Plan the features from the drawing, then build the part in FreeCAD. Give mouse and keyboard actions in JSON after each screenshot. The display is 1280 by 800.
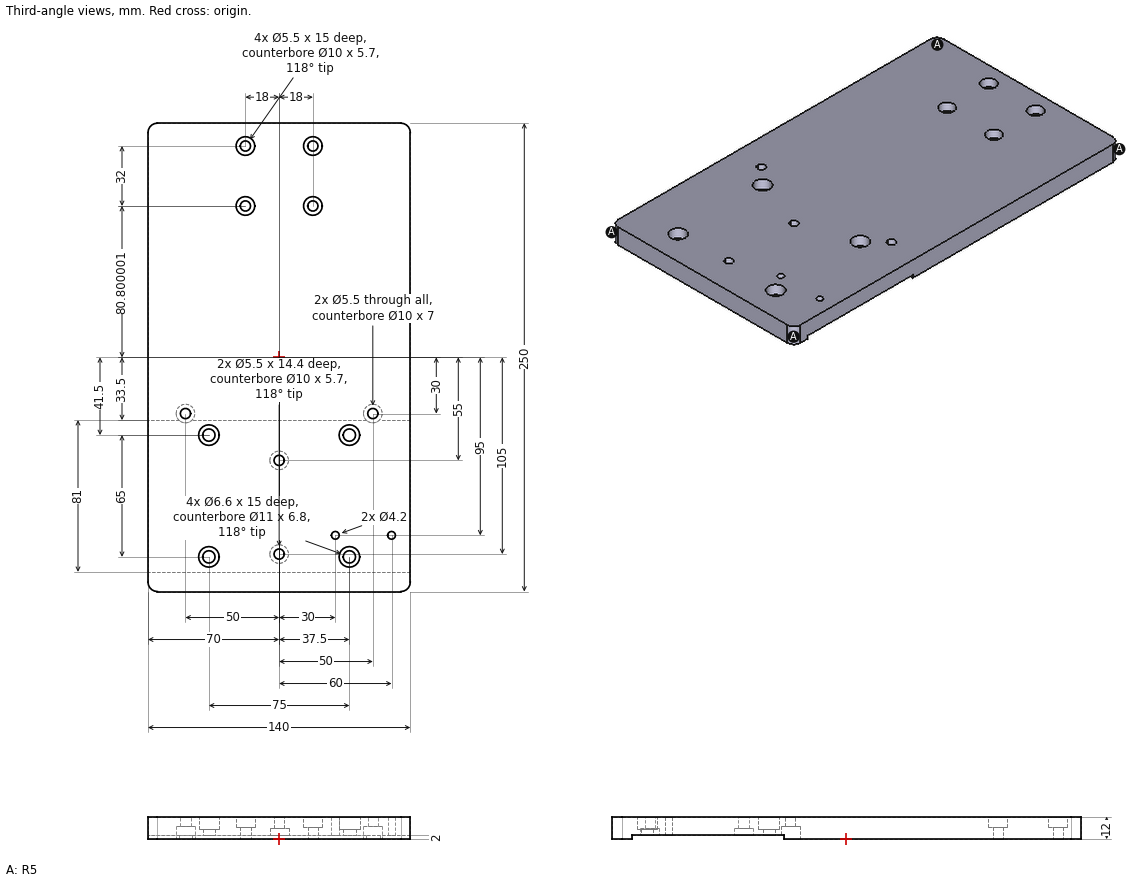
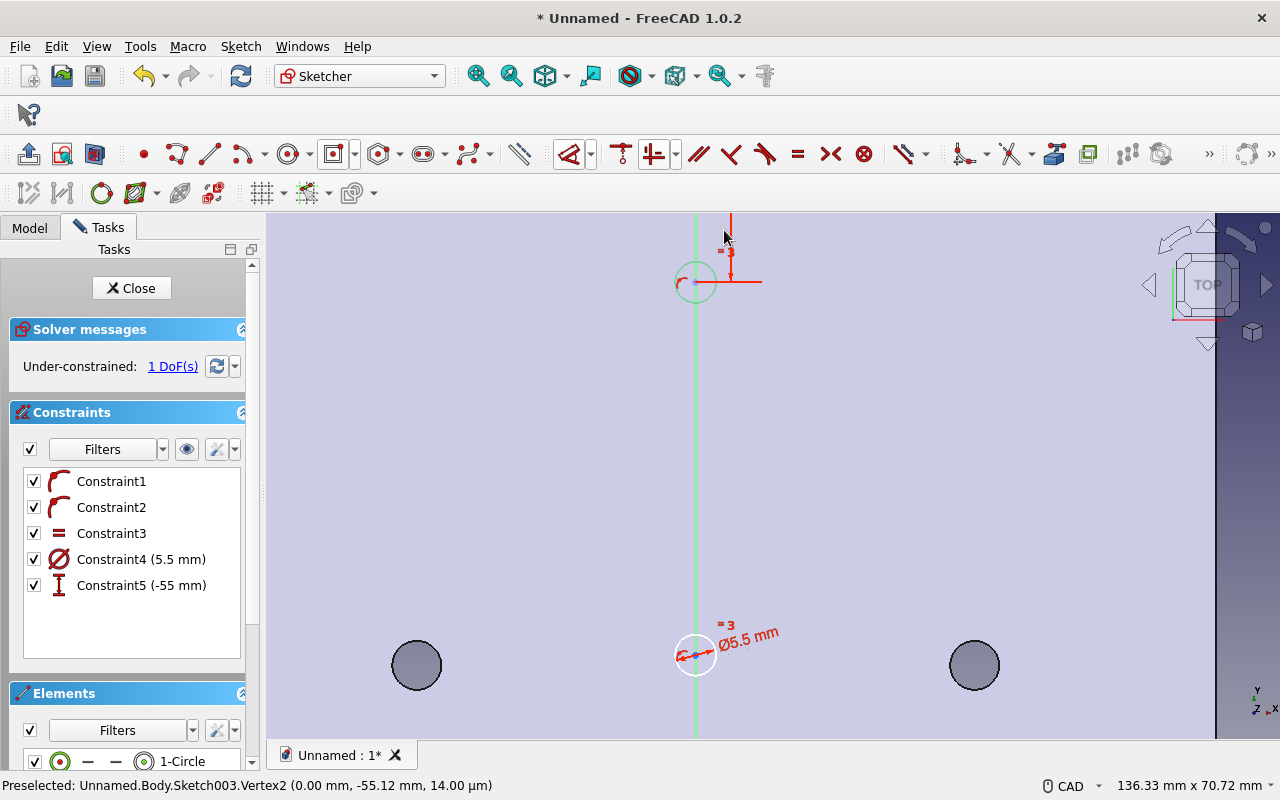
{"action": "left_click", "coordinate": [696, 655]}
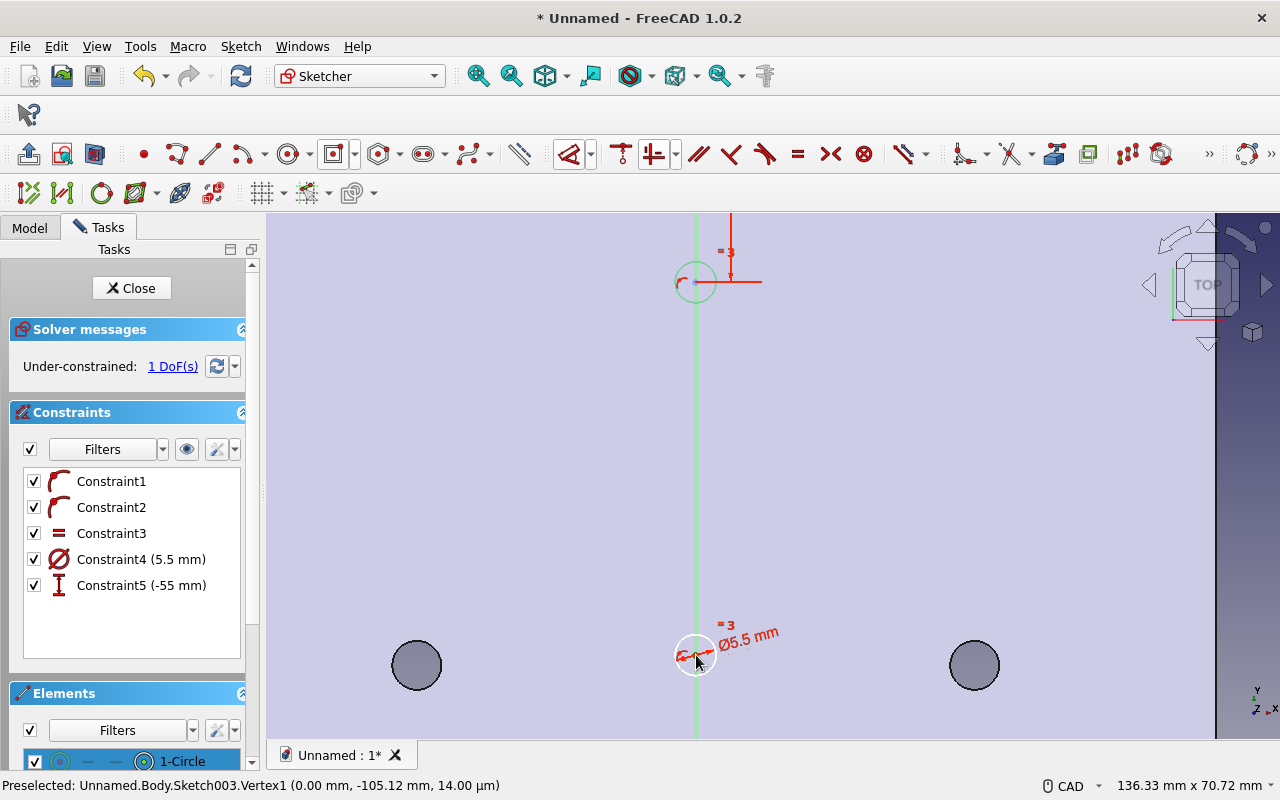
{"action": "key", "text": "i"}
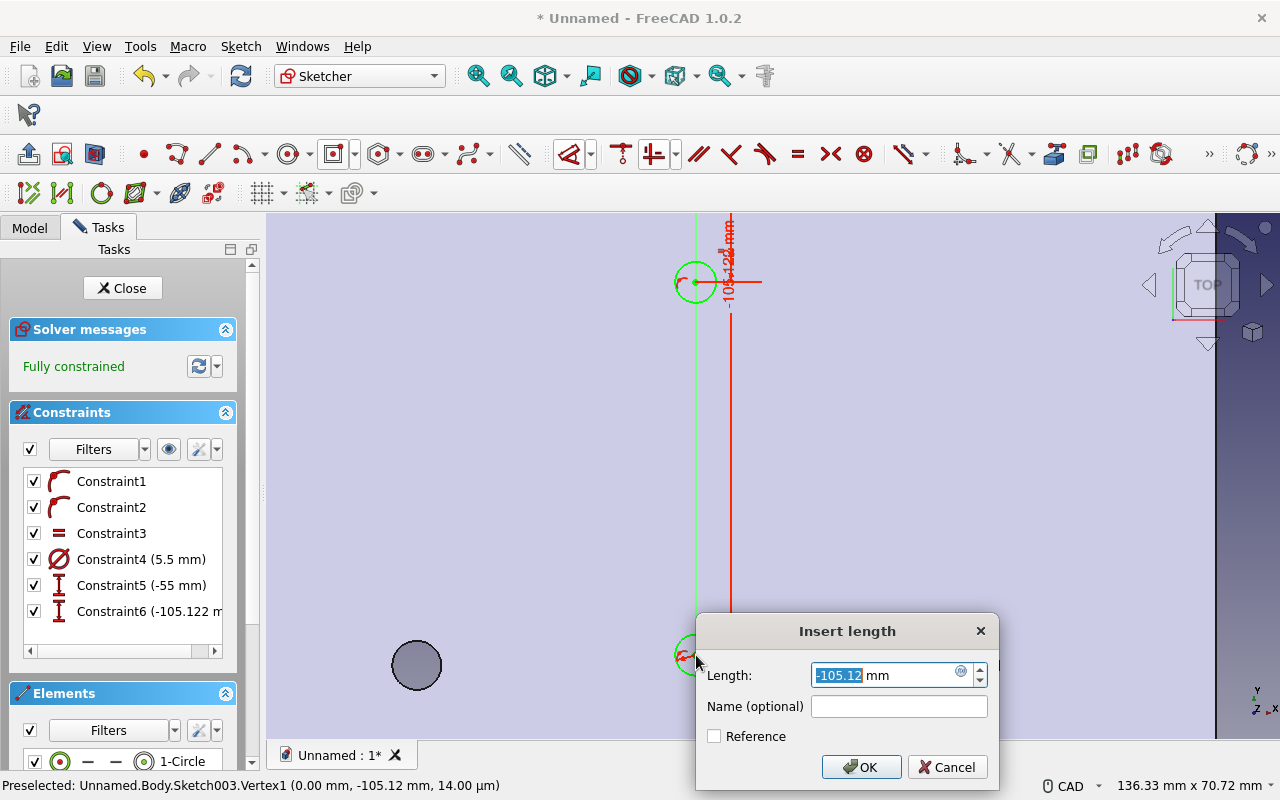
{"action": "type", "text": "-105"}
{"action": "key", "text": "Return"}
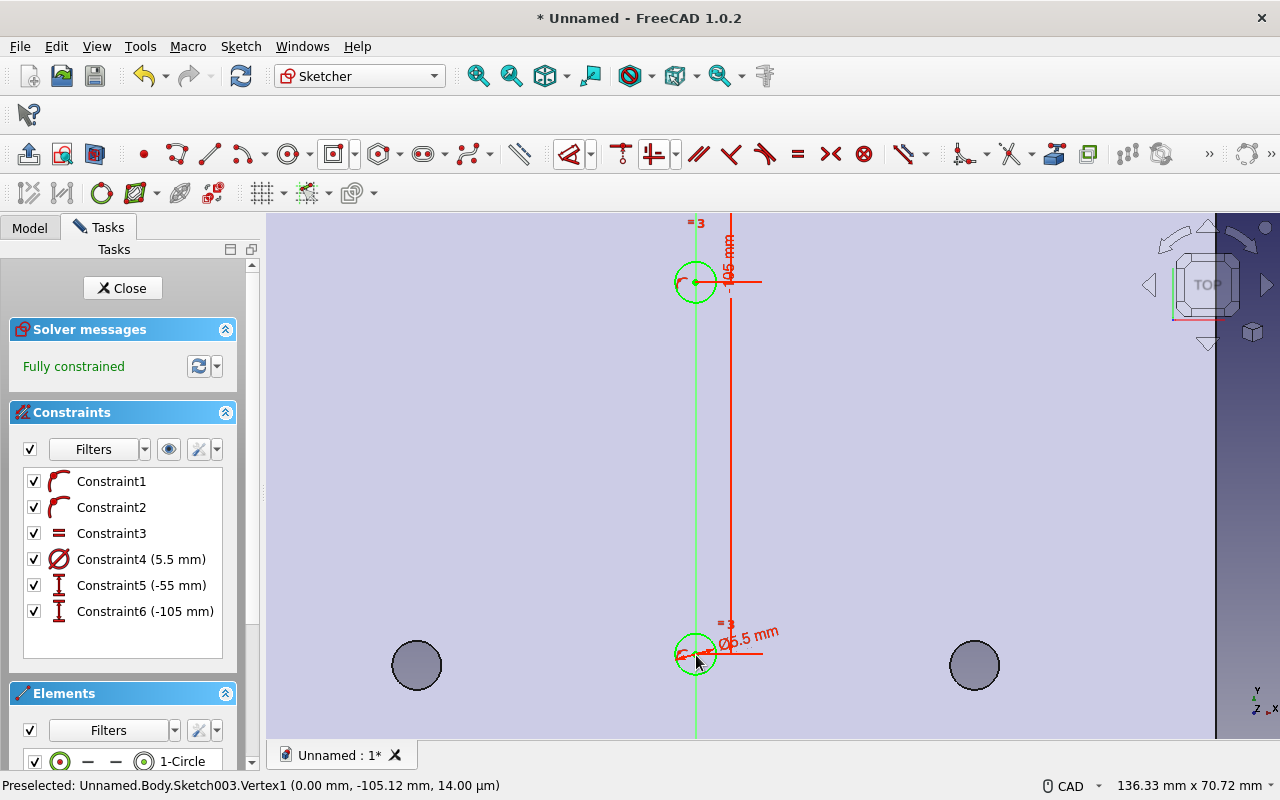
{"action": "left_click", "coordinate": [123, 288]}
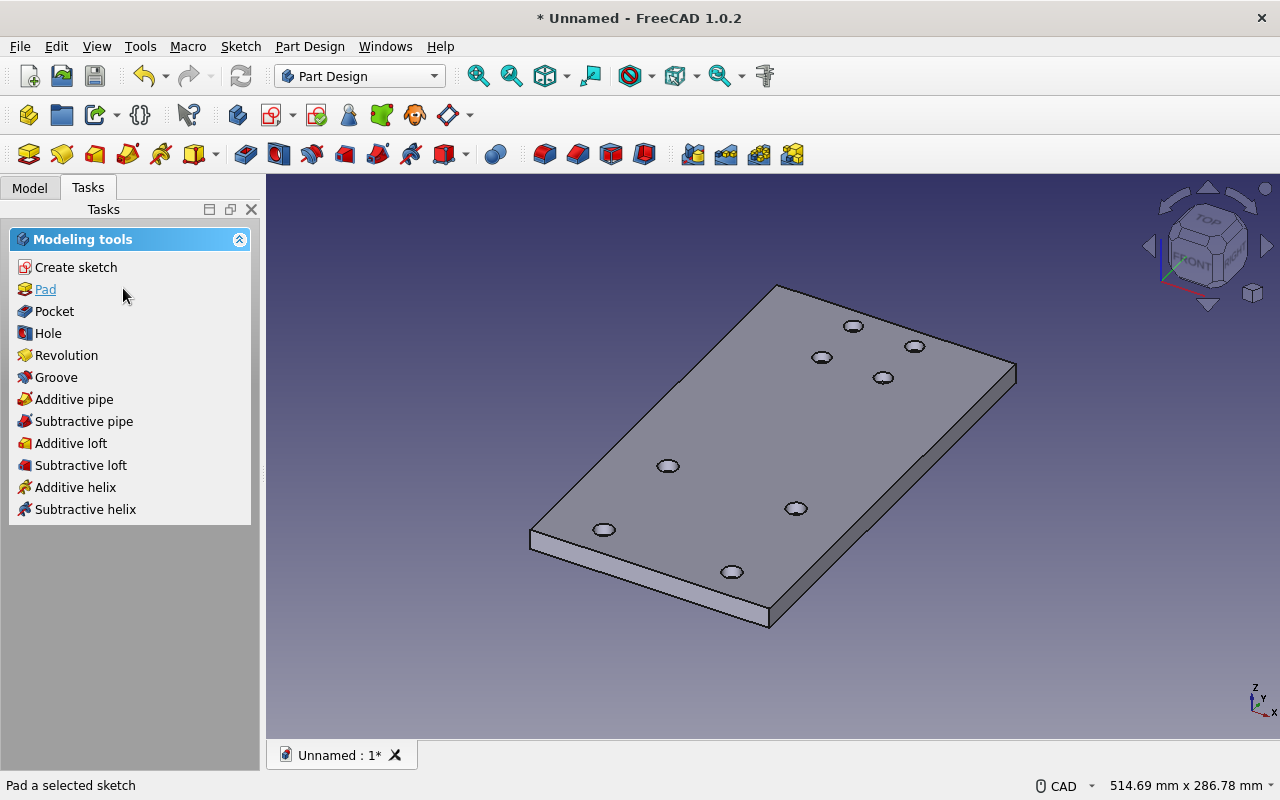
{"action": "left_click", "coordinate": [279, 154]}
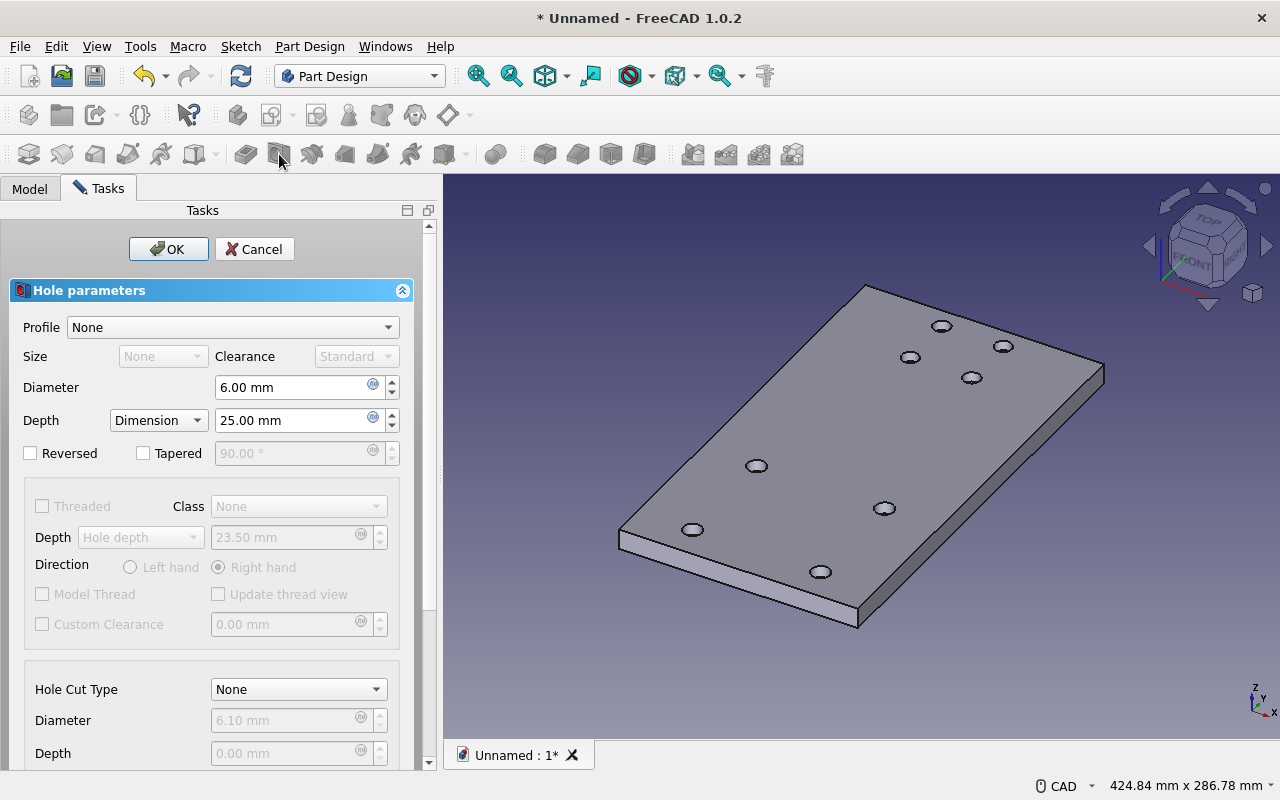
{"action": "triple_click", "coordinate": [300, 388]}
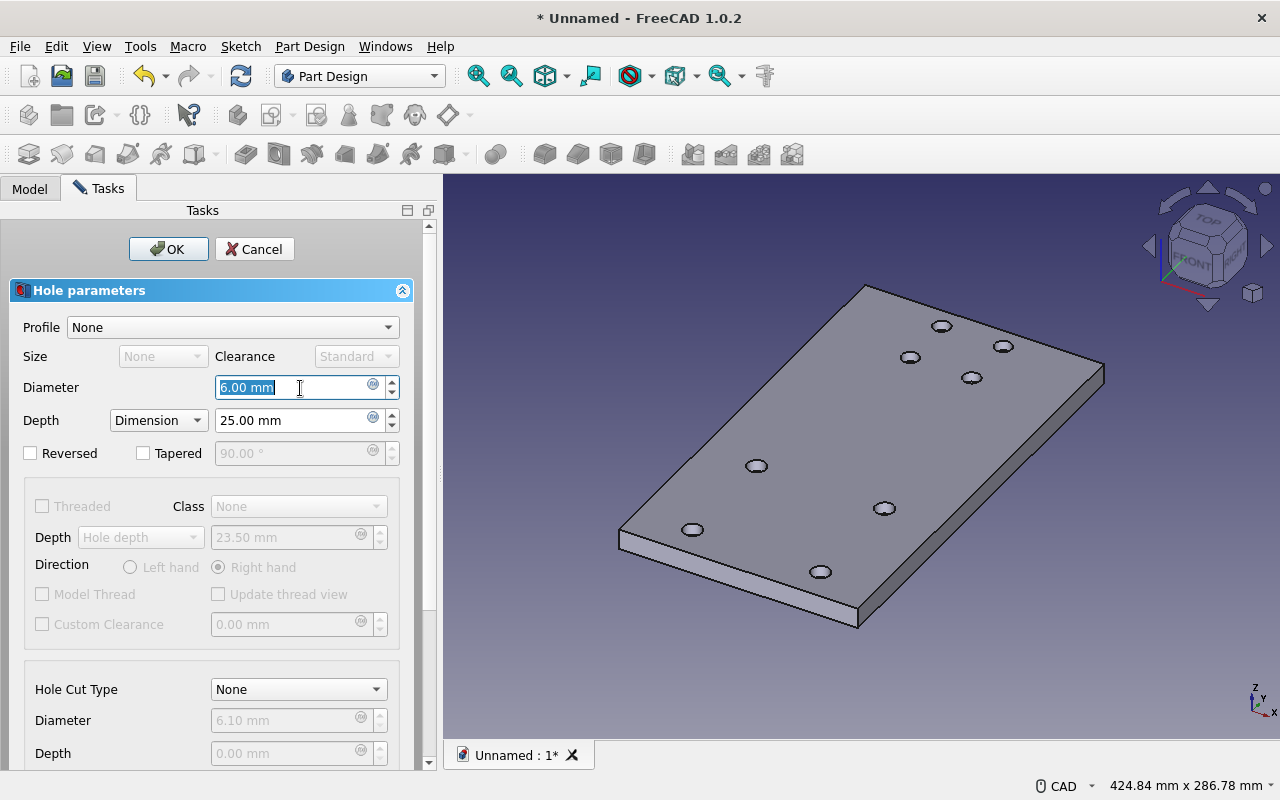
{"action": "type", "text": "5.5"}
{"action": "key", "text": "Tab"}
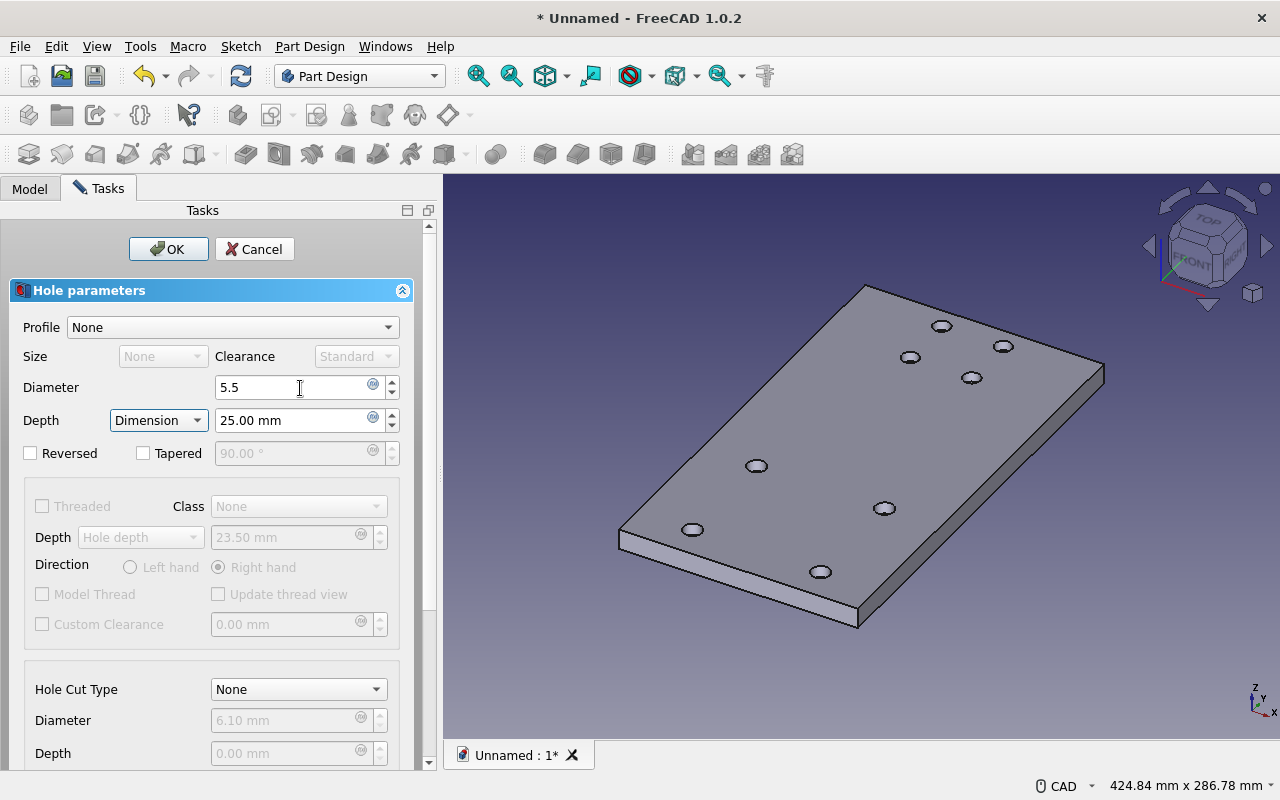
{"action": "triple_click", "coordinate": [300, 420]}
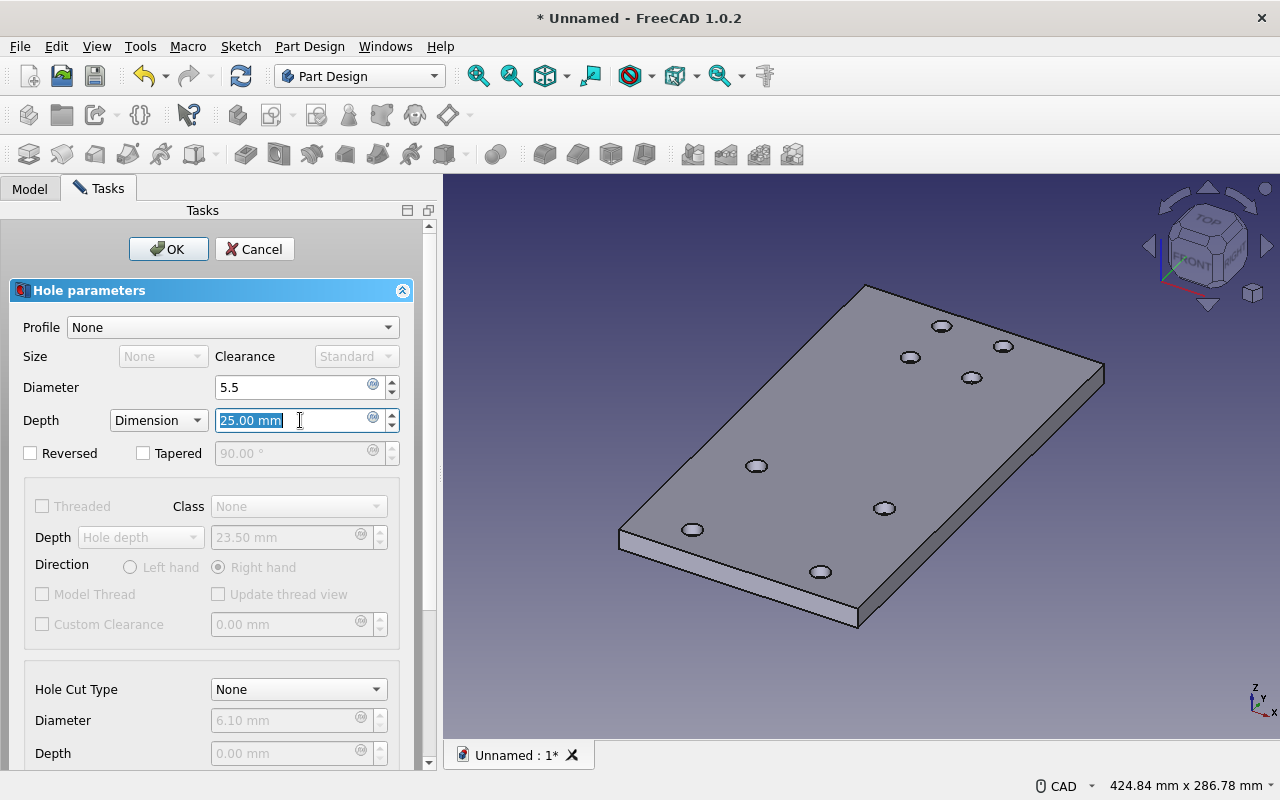
{"action": "type", "text": "14.4"}
{"action": "key", "text": "Tab"}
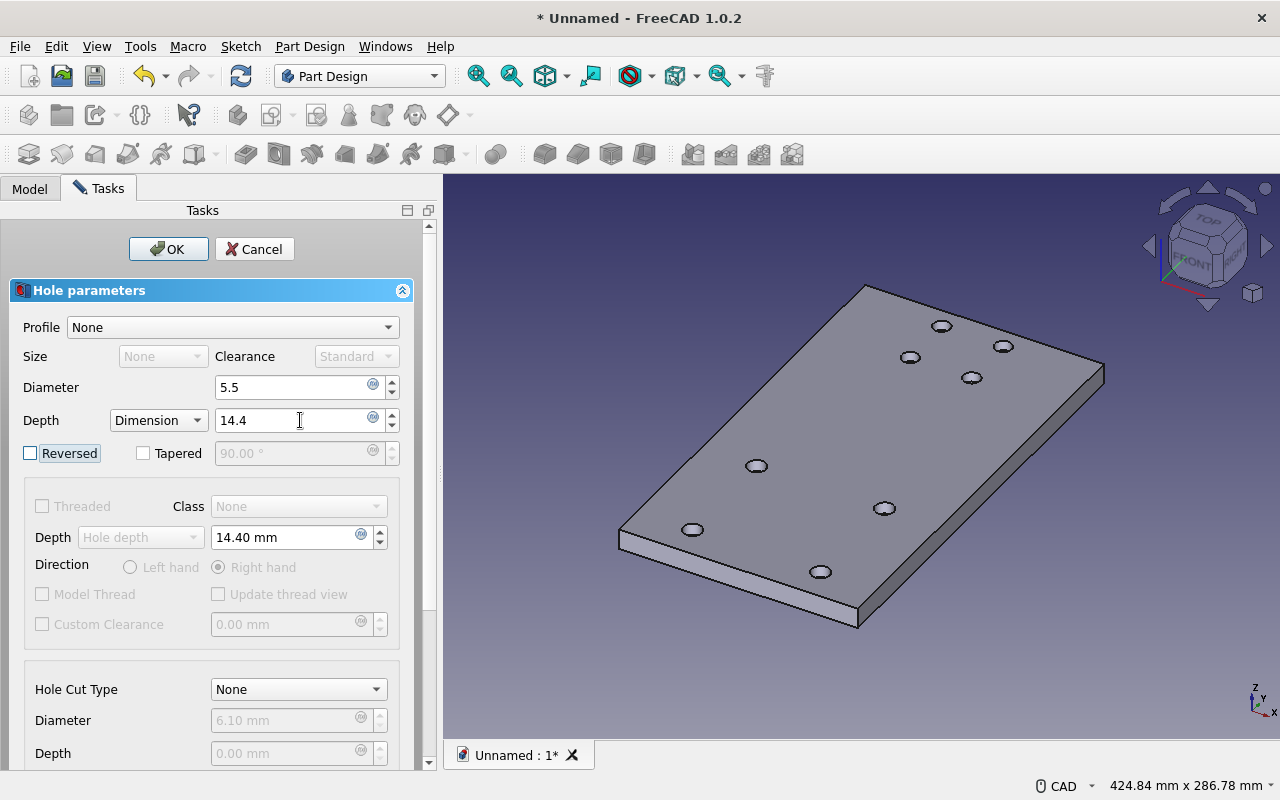
{"action": "left_click", "coordinate": [31, 453]}